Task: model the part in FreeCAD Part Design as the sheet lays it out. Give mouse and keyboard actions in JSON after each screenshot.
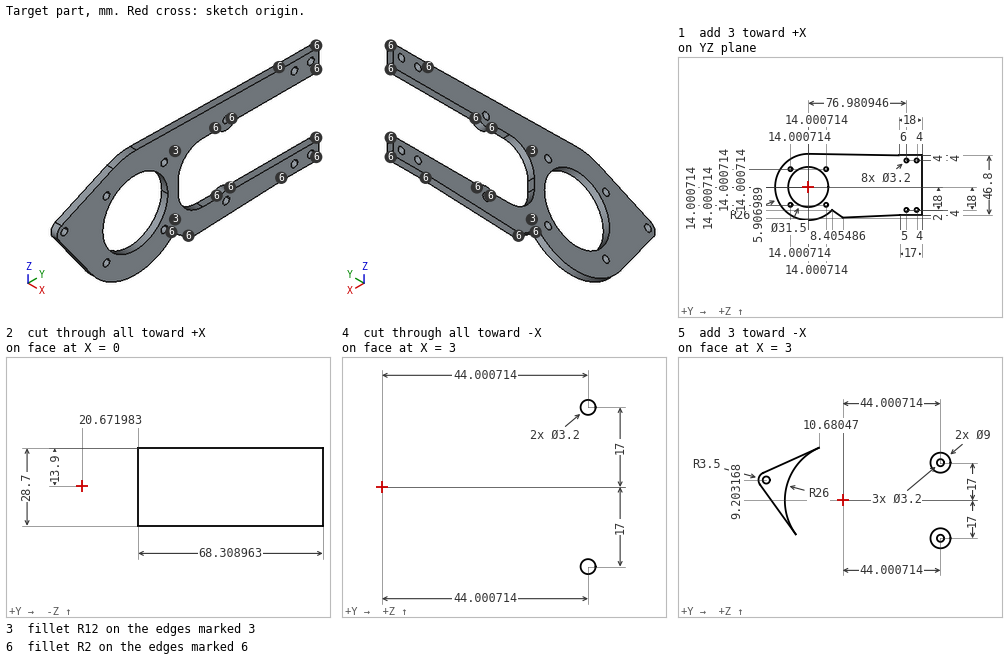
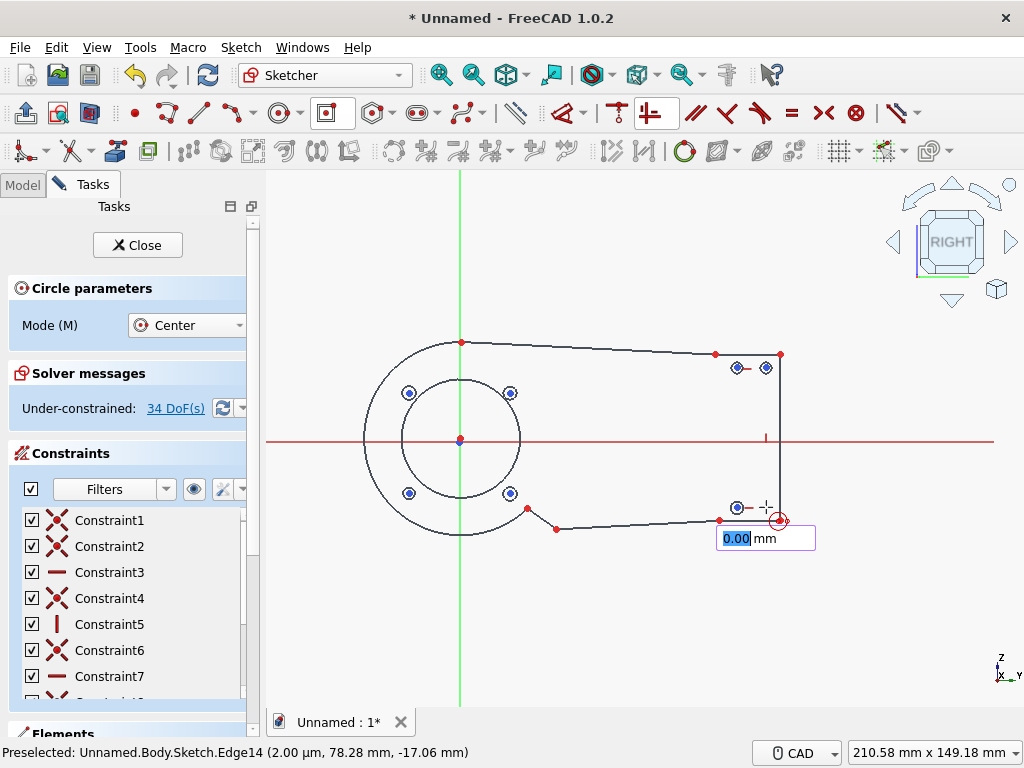
{"action": "scroll", "coordinate": [762, 503], "scroll_direction": "up", "scroll_amount": 6}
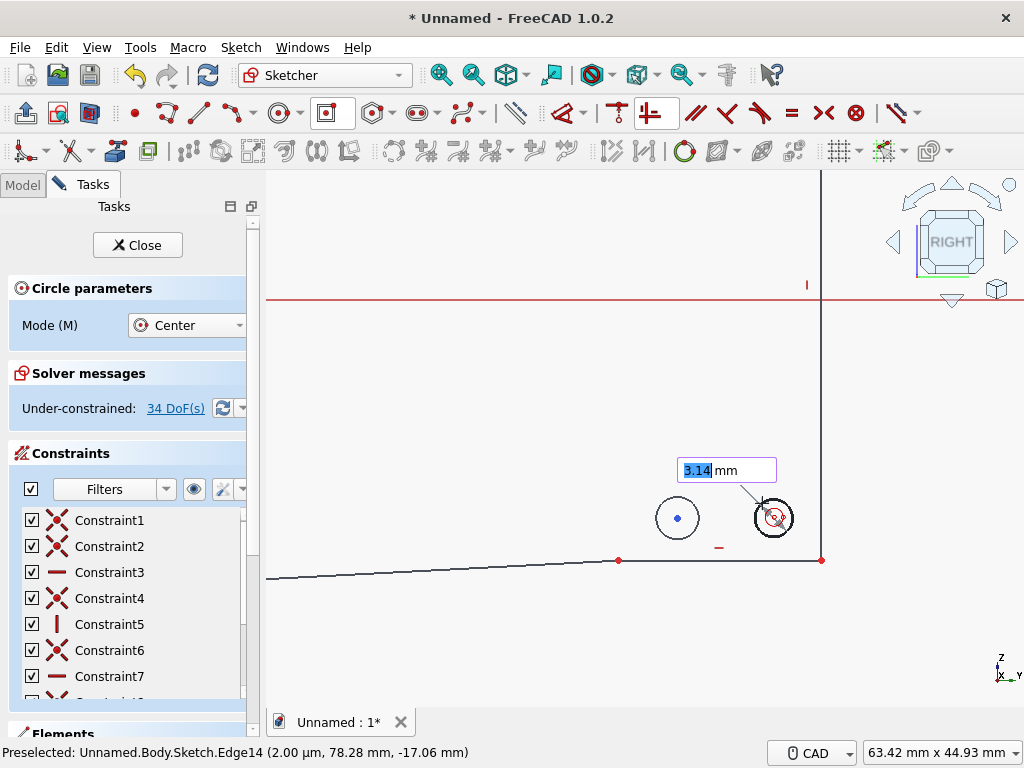
{"action": "left_click", "coordinate": [760, 501]}
{"action": "key", "text": "Escape"}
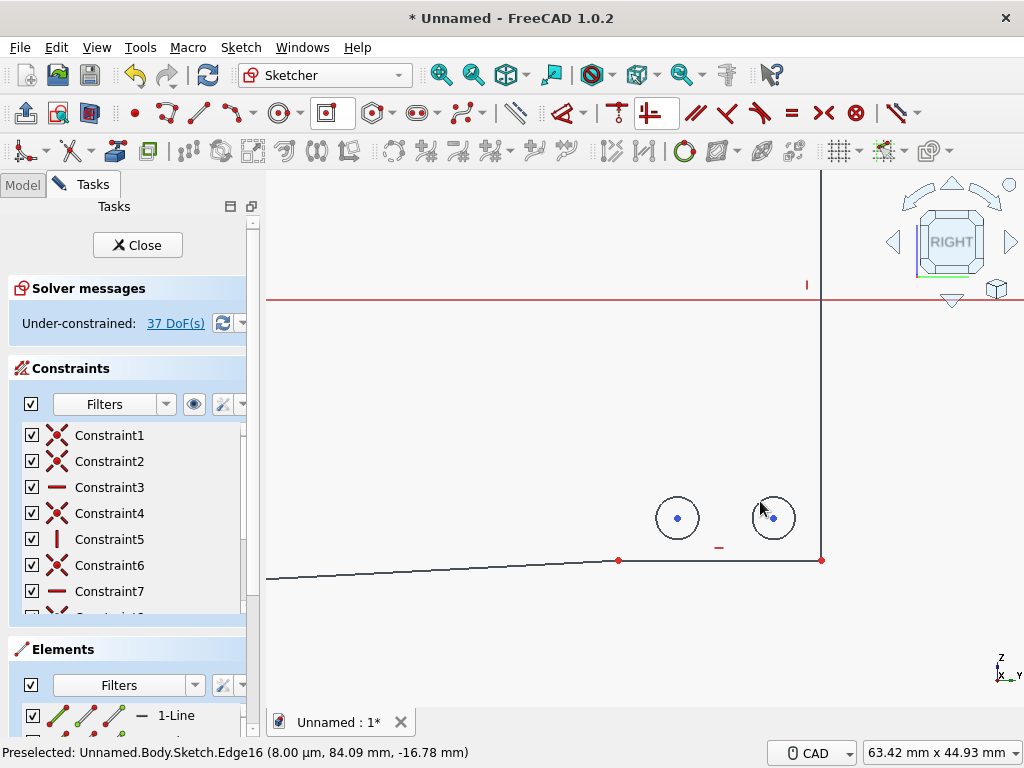
{"action": "scroll", "coordinate": [762, 503], "scroll_direction": "down", "scroll_amount": 6}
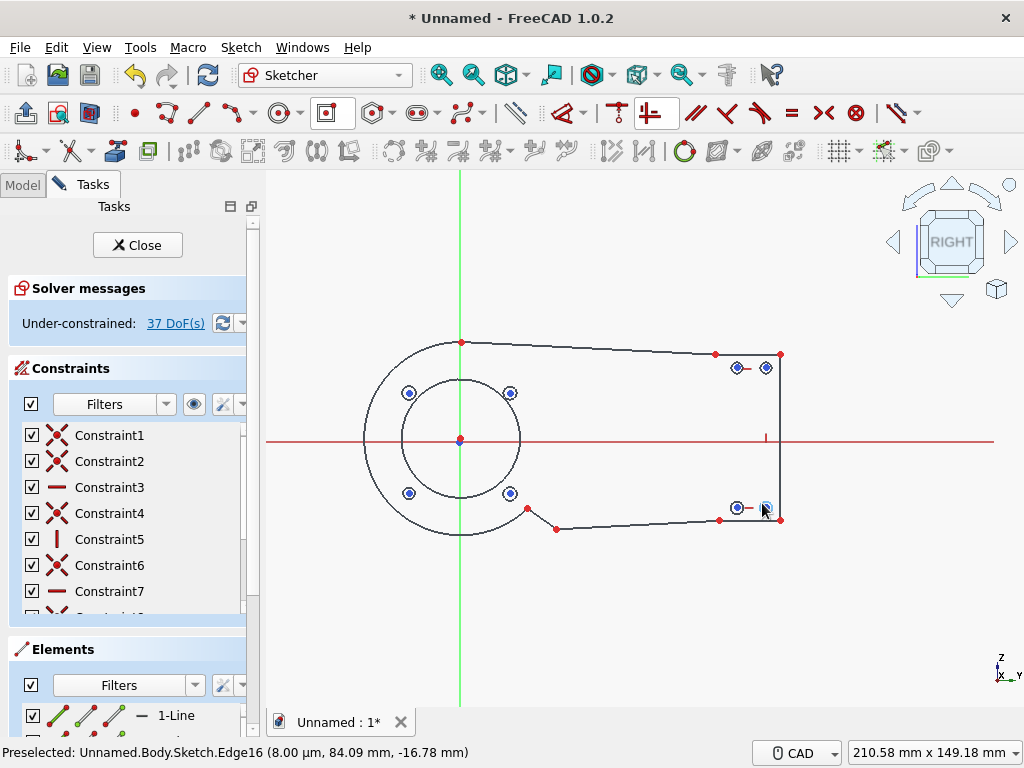
{"action": "left_click", "coordinate": [639, 351]}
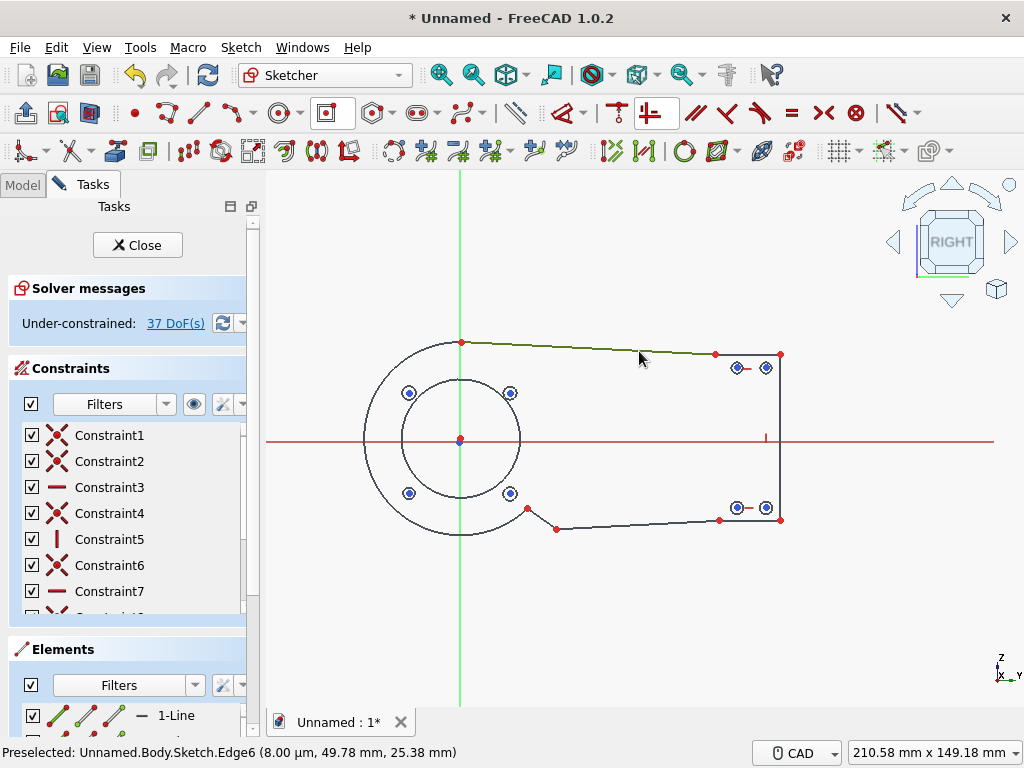
{"action": "left_click", "coordinate": [372, 401]}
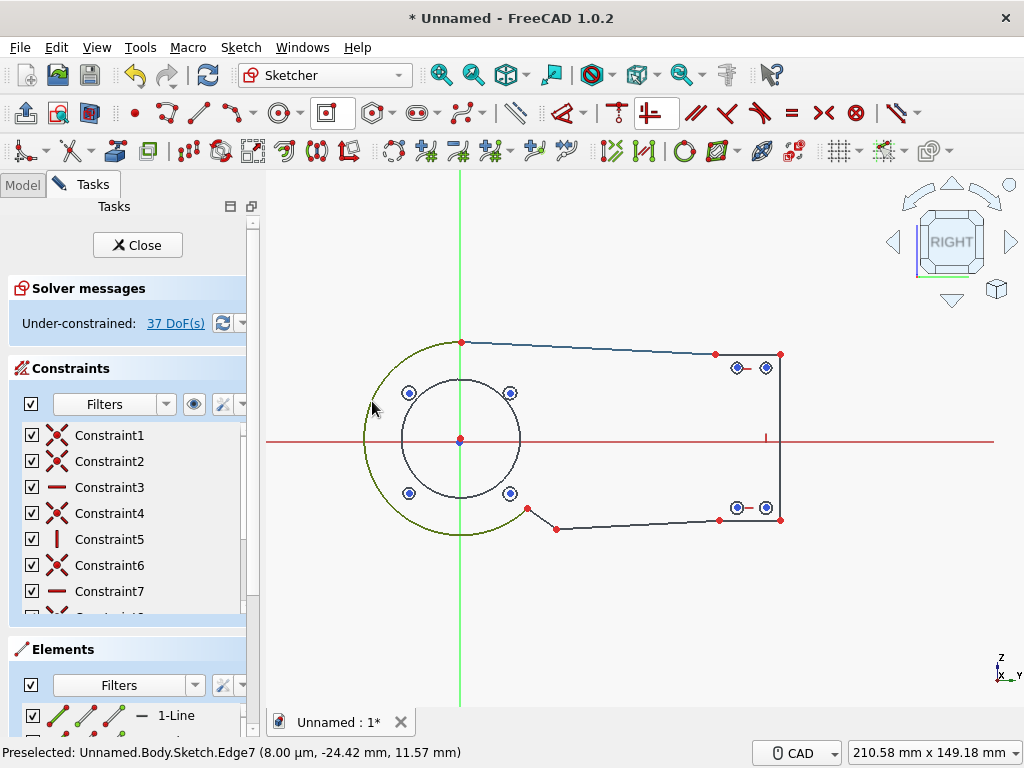
{"action": "left_click", "coordinate": [760, 114]}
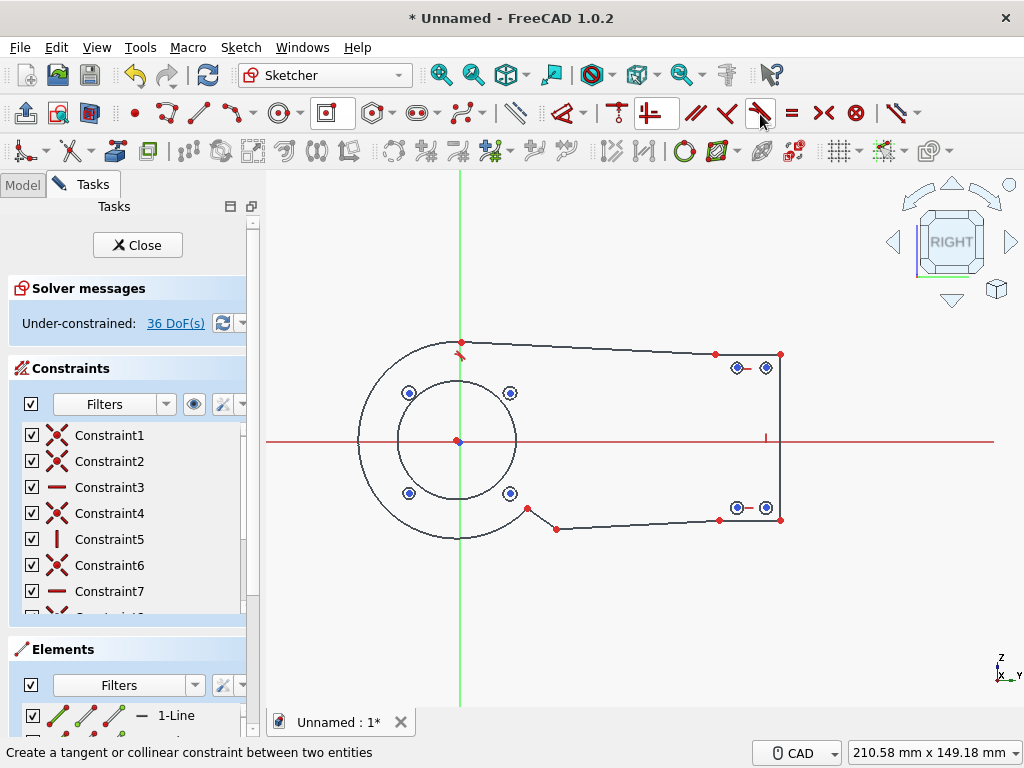
{"action": "scroll", "coordinate": [458, 441], "scroll_direction": "up", "scroll_amount": 10}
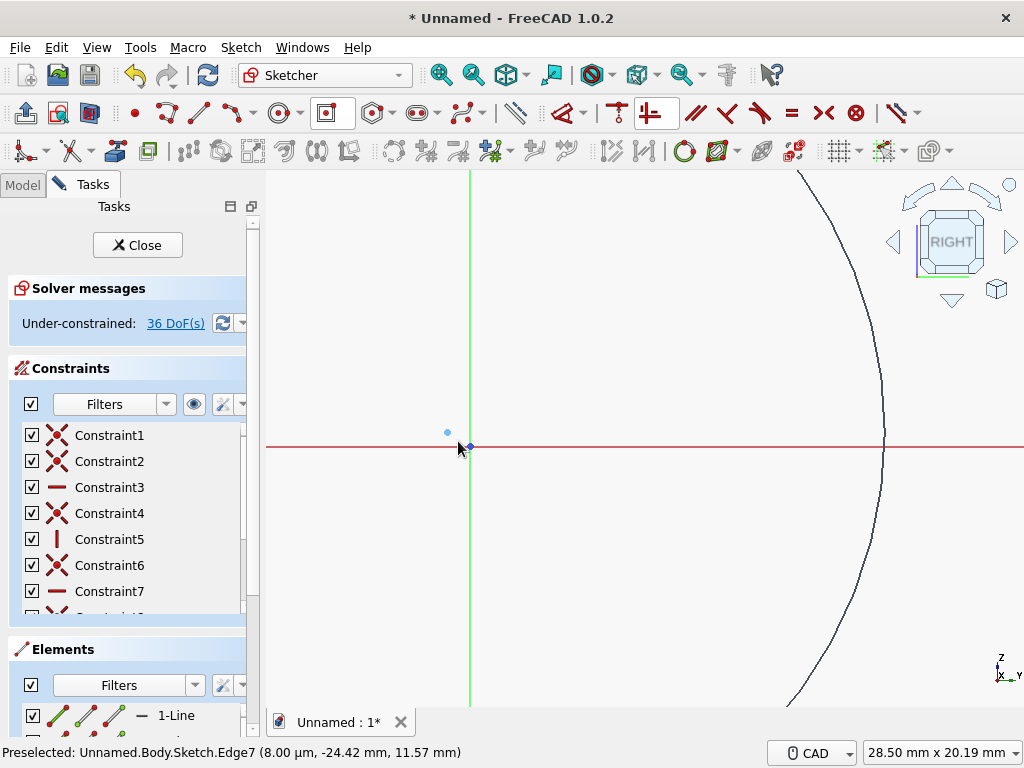
{"action": "left_click_drag", "start_coordinate": [437, 422], "coordinate": [480, 457]}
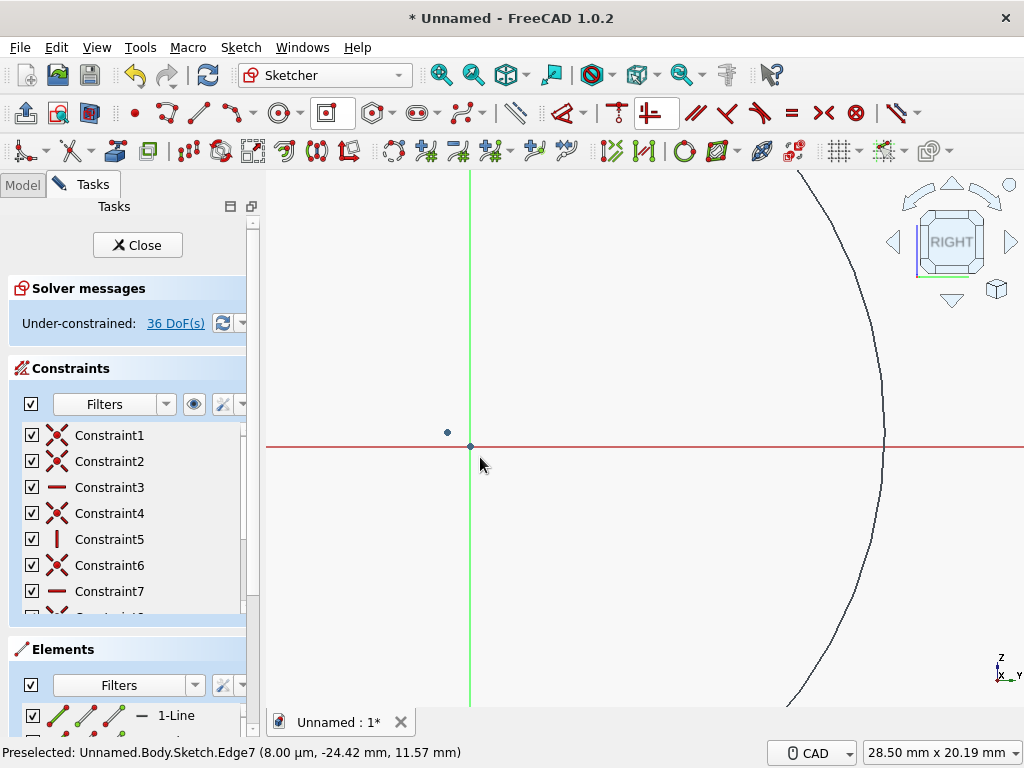
{"action": "left_click", "coordinate": [618, 114]}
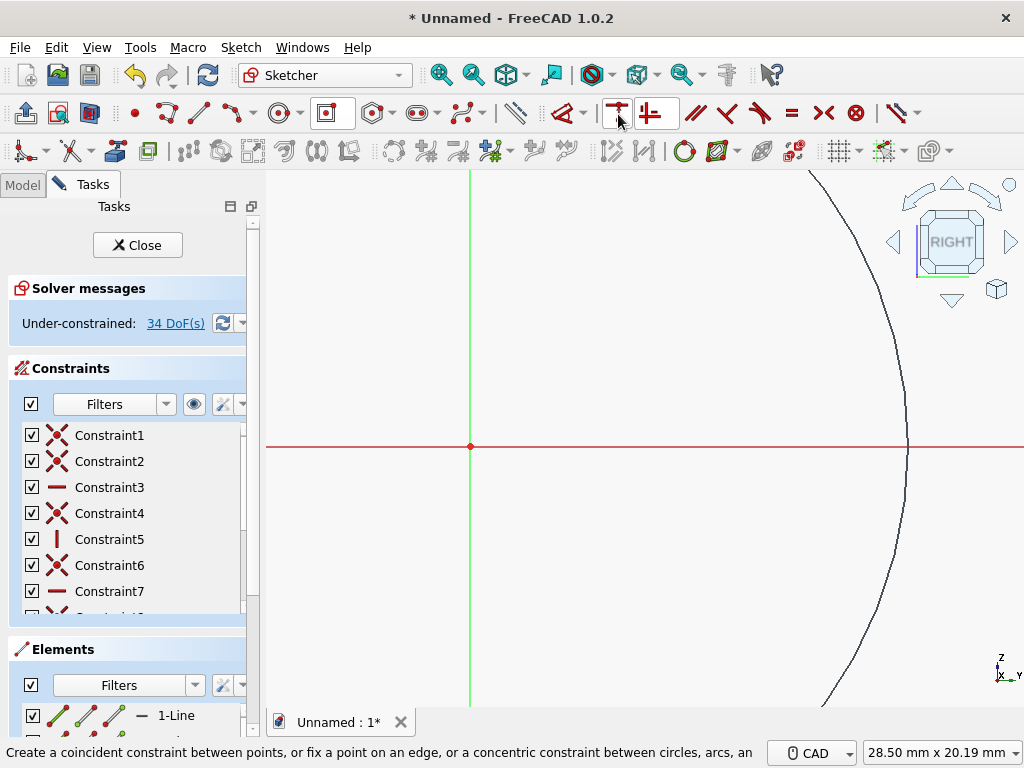
{"action": "scroll", "coordinate": [458, 441], "scroll_direction": "down", "scroll_amount": 10}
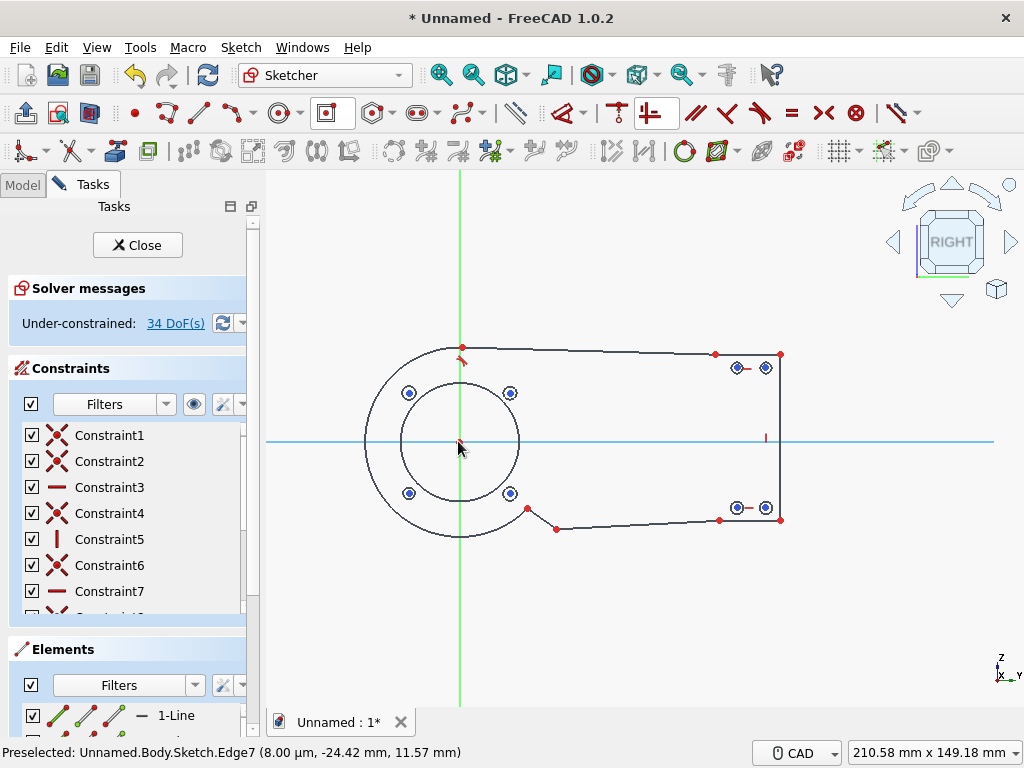
{"action": "scroll", "coordinate": [414, 388], "scroll_direction": "up", "scroll_amount": 4}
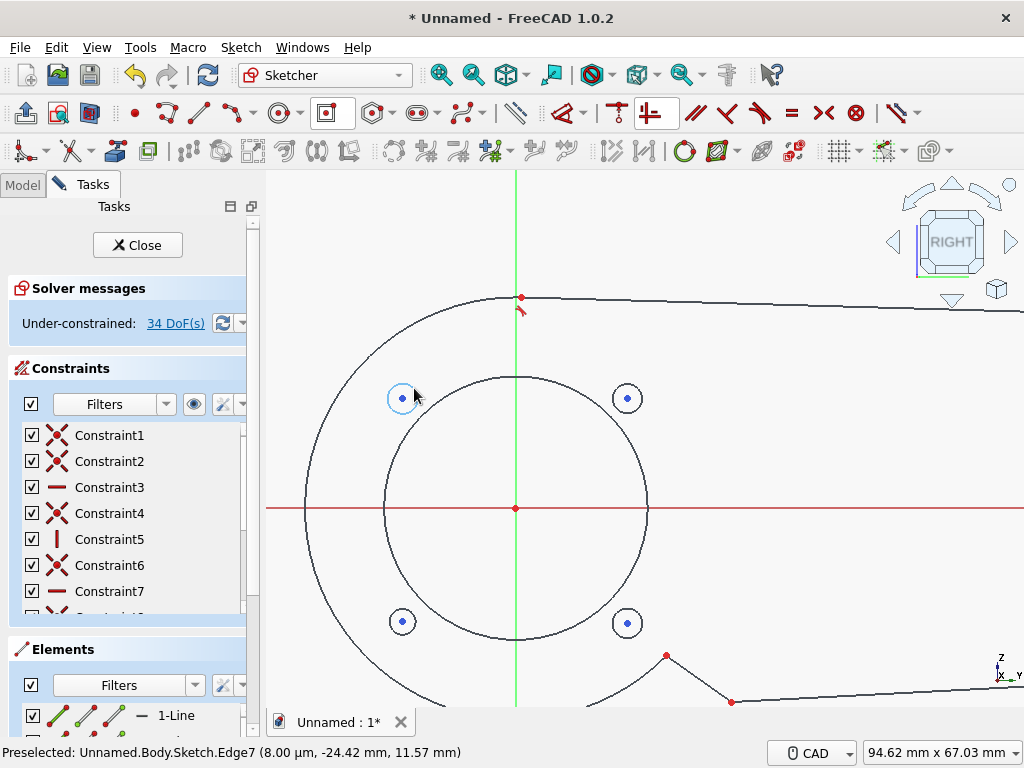
{"action": "left_click", "coordinate": [413, 388]}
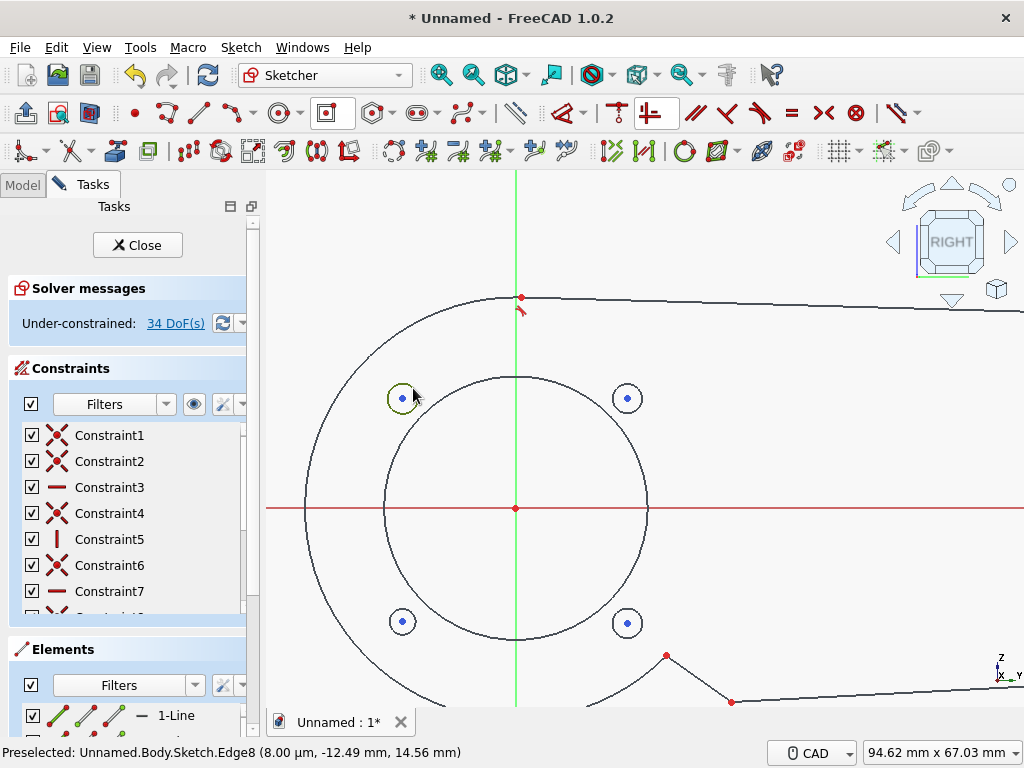
{"action": "left_click", "coordinate": [638, 388]}